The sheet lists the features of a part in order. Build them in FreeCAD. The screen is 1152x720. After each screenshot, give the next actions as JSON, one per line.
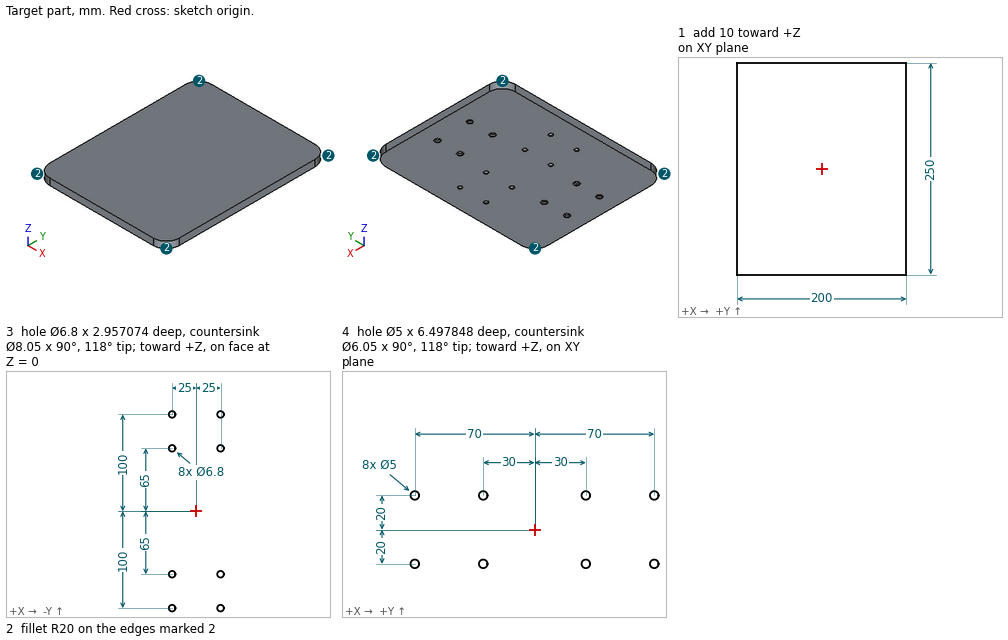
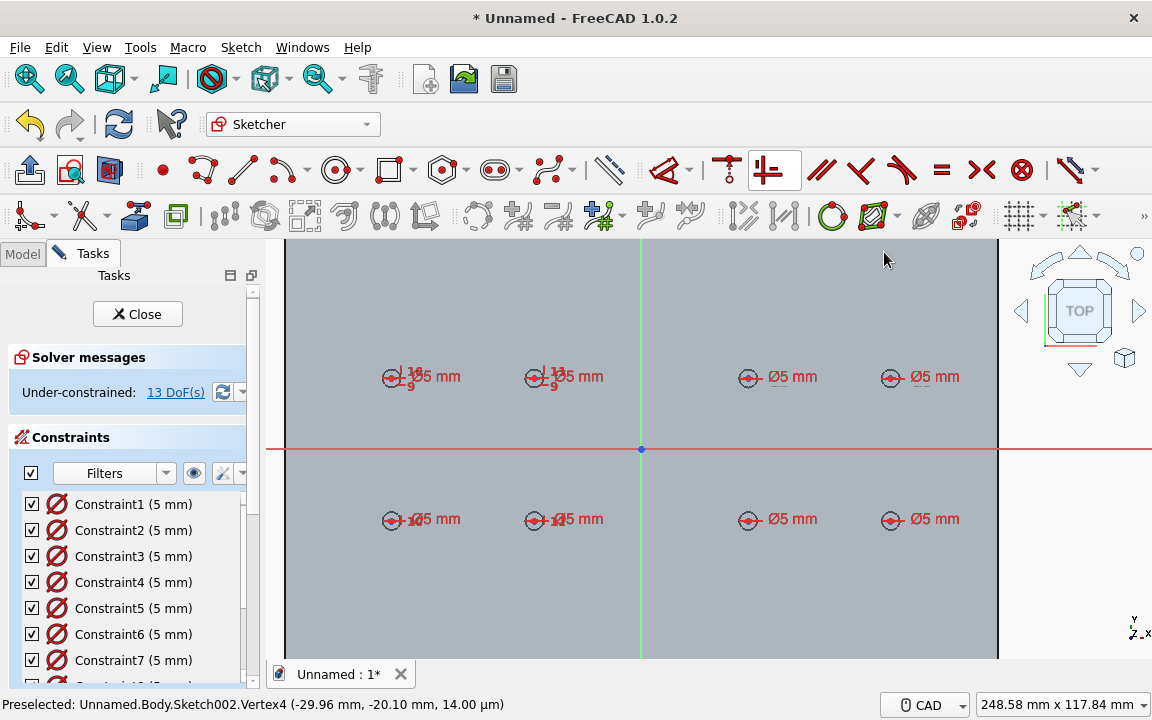
{"action": "left_click", "coordinate": [392, 521]}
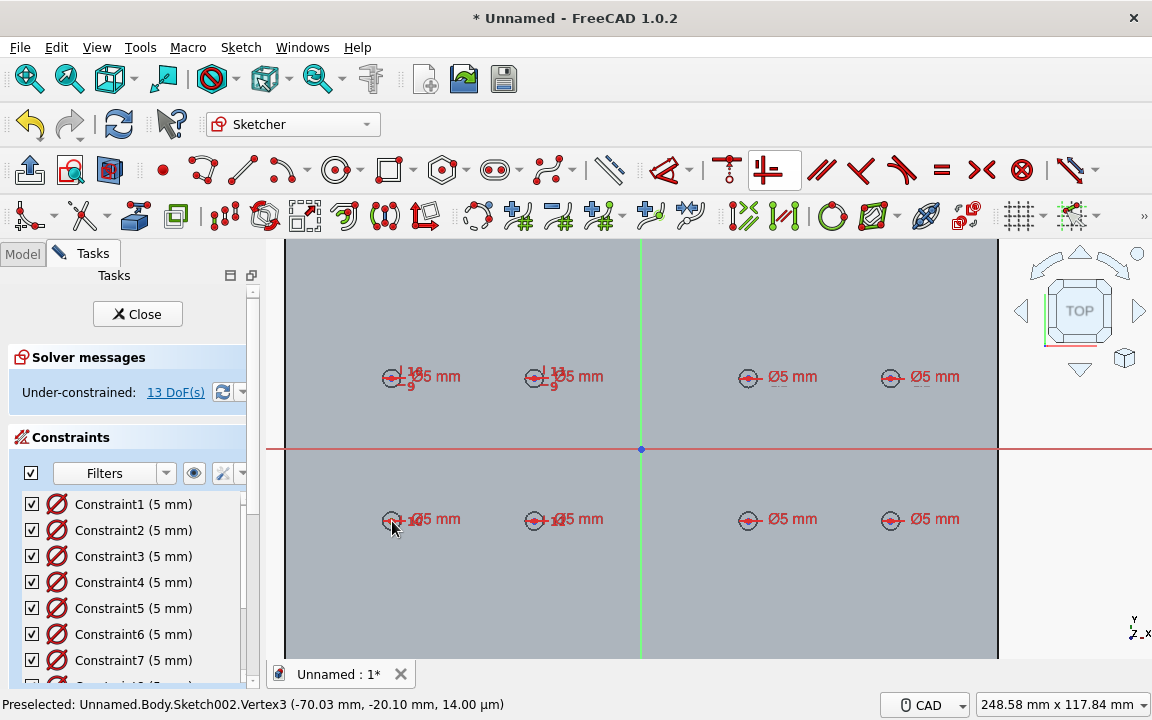
{"action": "left_click", "coordinate": [534, 521]}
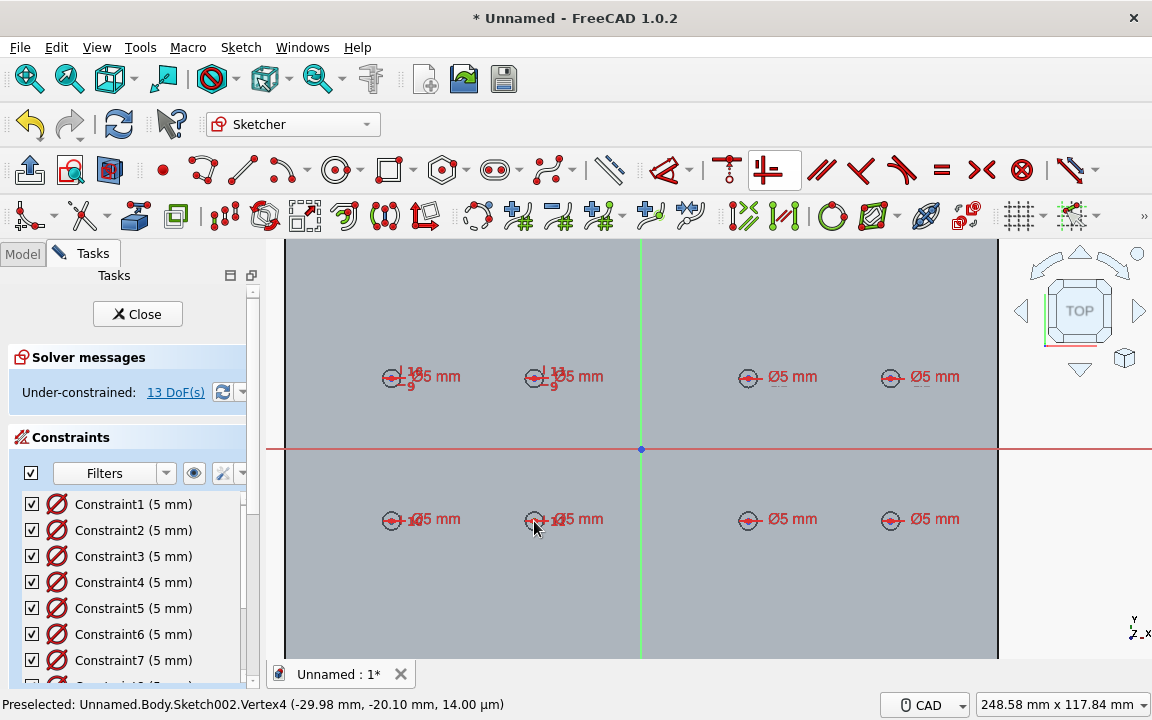
{"action": "key", "text": "h"}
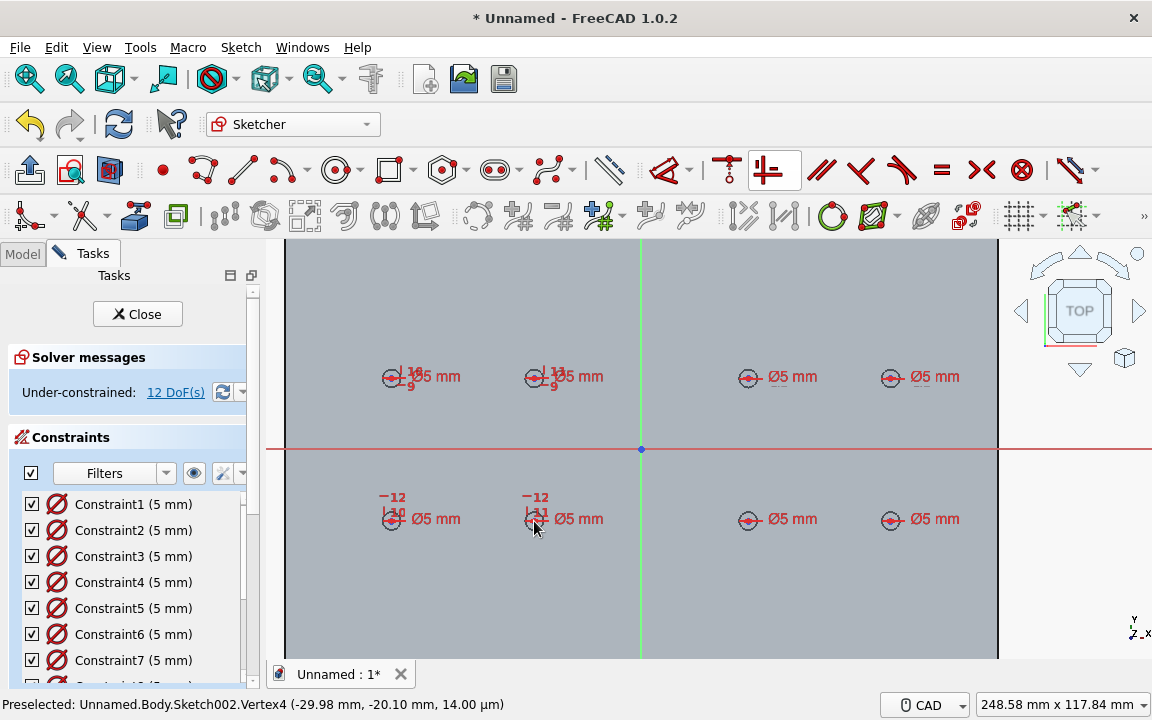
{"action": "left_click", "coordinate": [534, 378]}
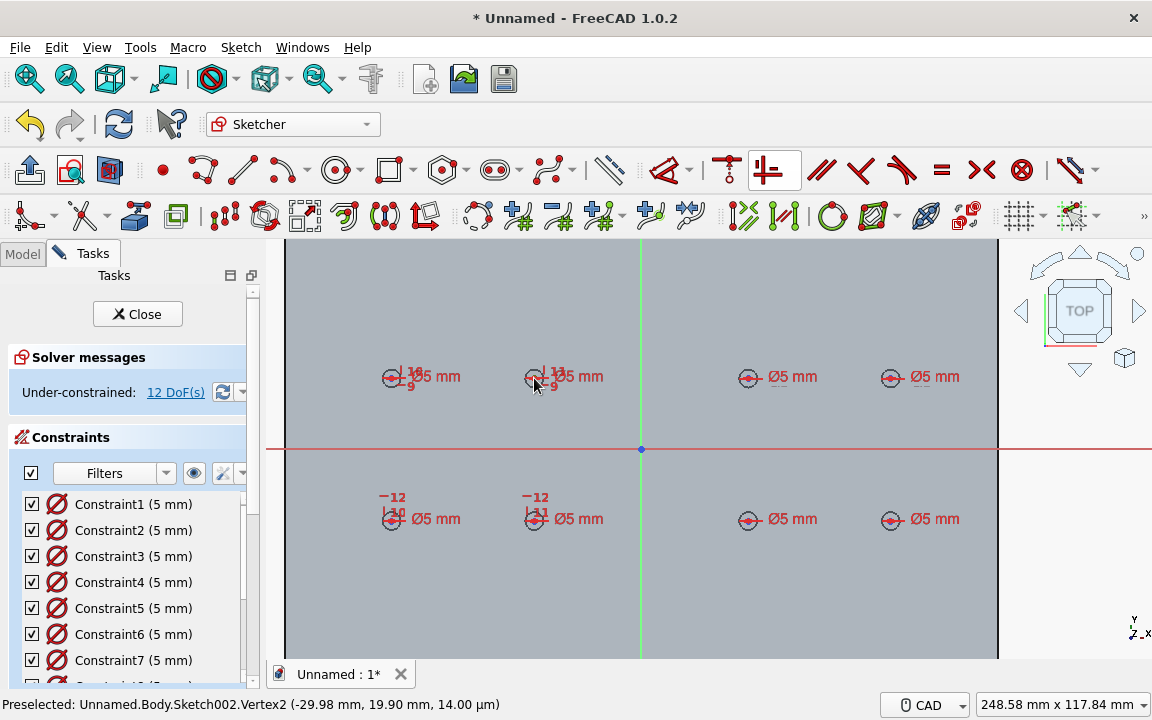
{"action": "left_click", "coordinate": [748, 379]}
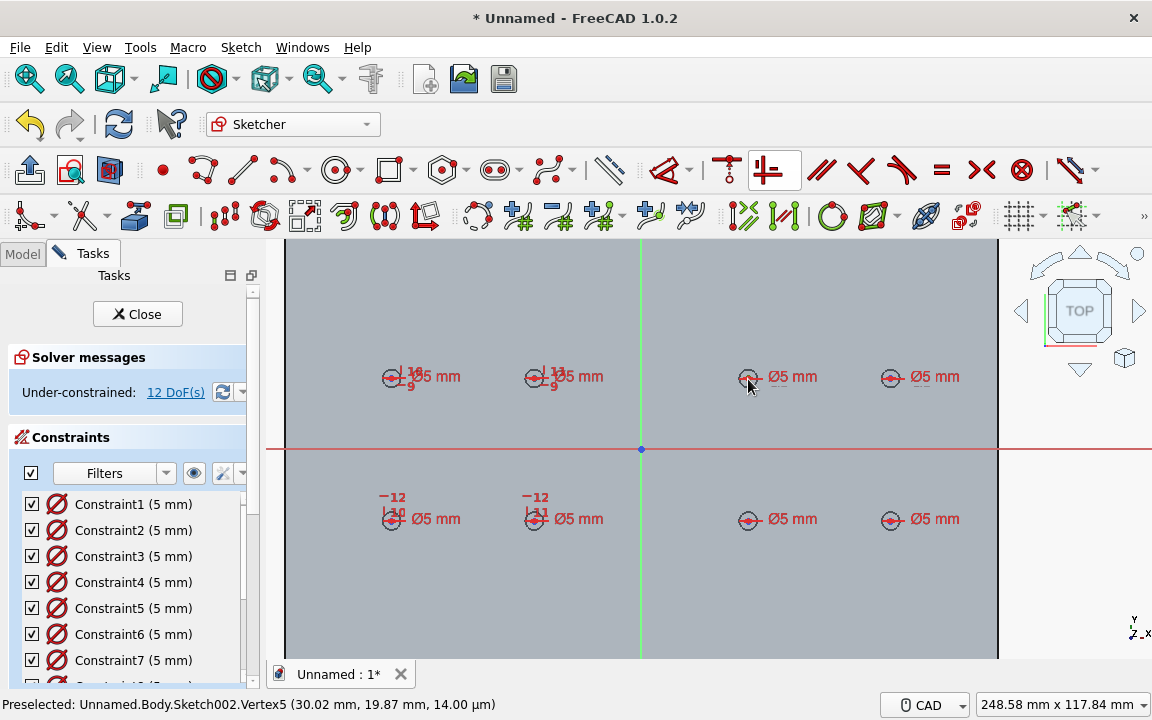
{"action": "key", "text": "h"}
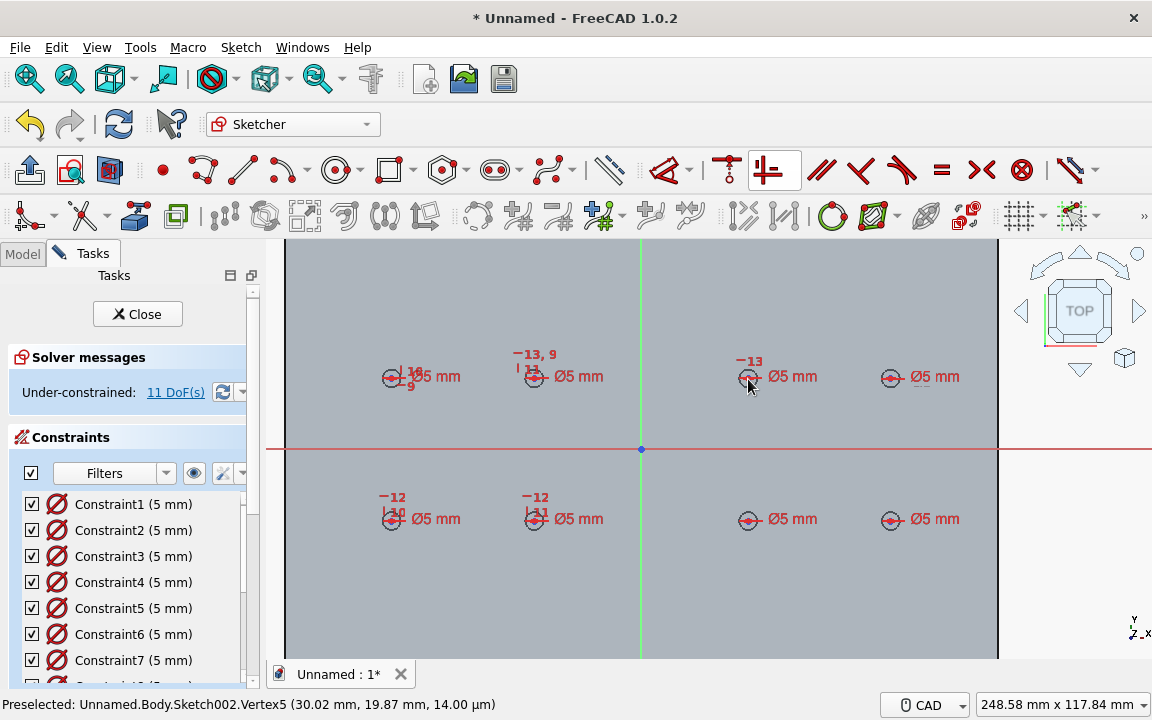
{"action": "left_click", "coordinate": [748, 378]}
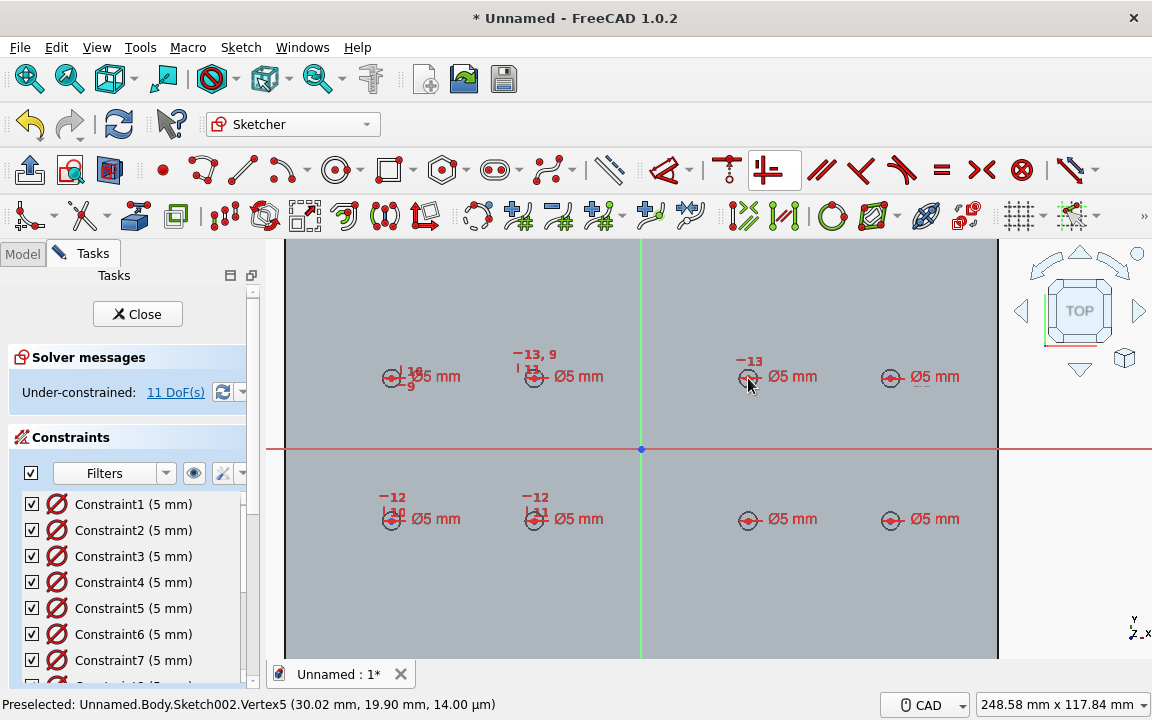
{"action": "left_click", "coordinate": [748, 521]}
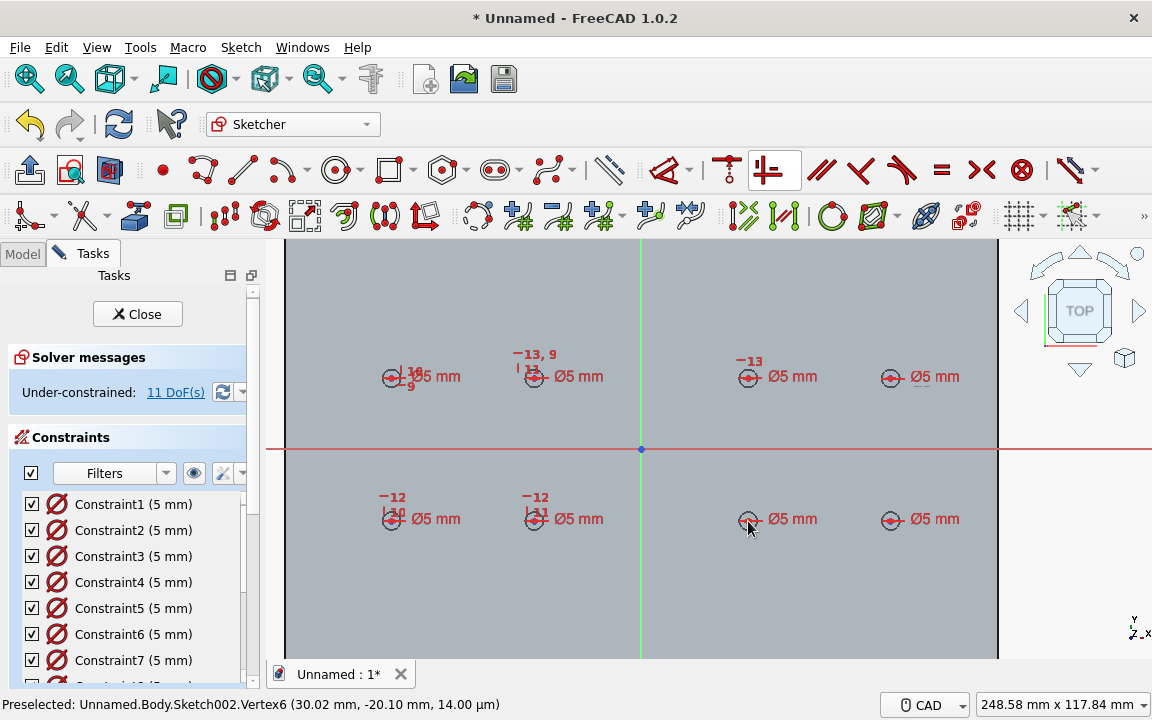
{"action": "key", "text": "v"}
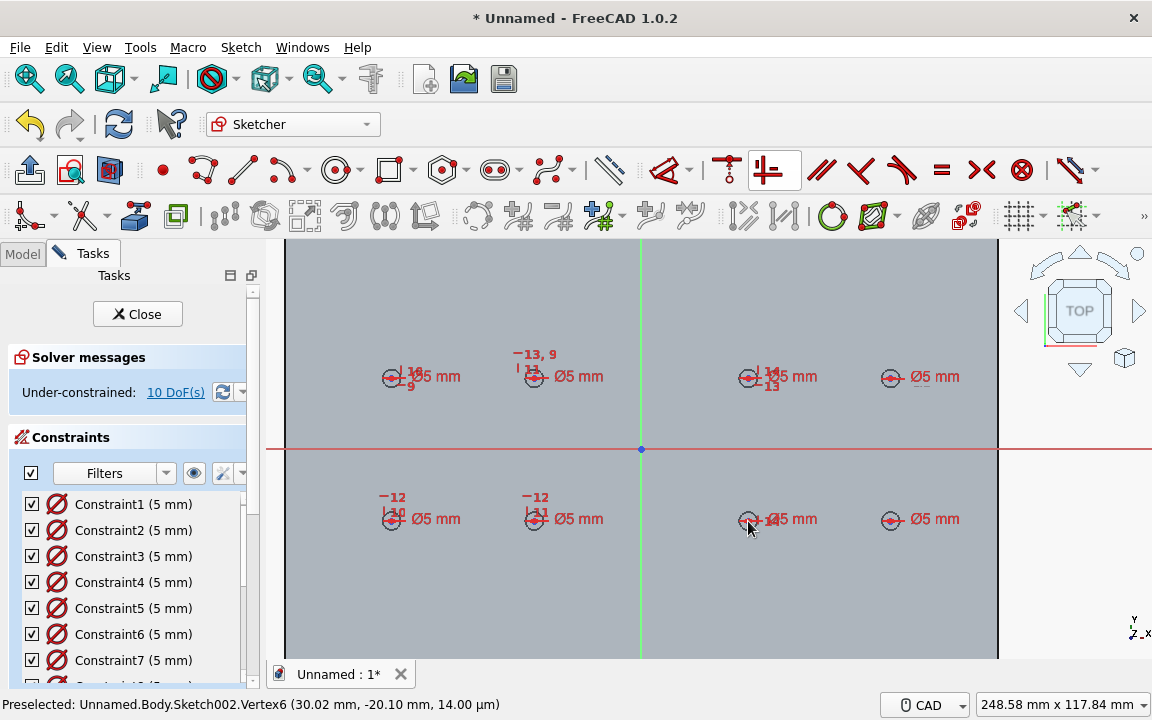
{"action": "left_click", "coordinate": [534, 521]}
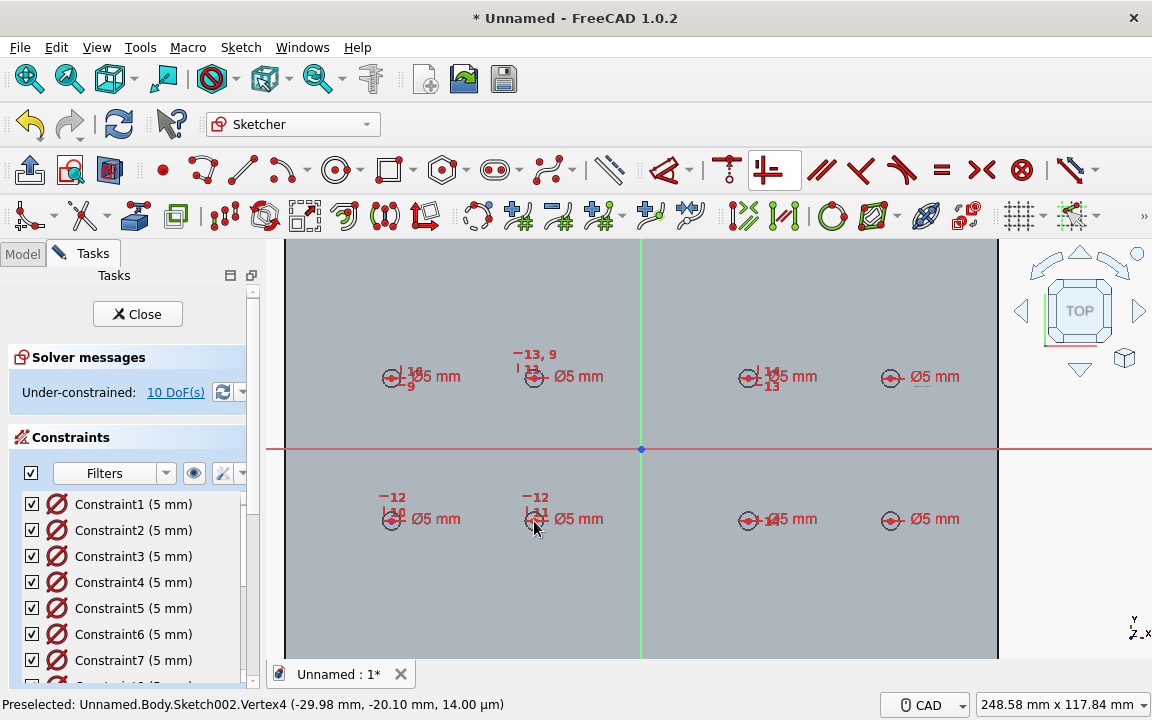
{"action": "left_click", "coordinate": [748, 521]}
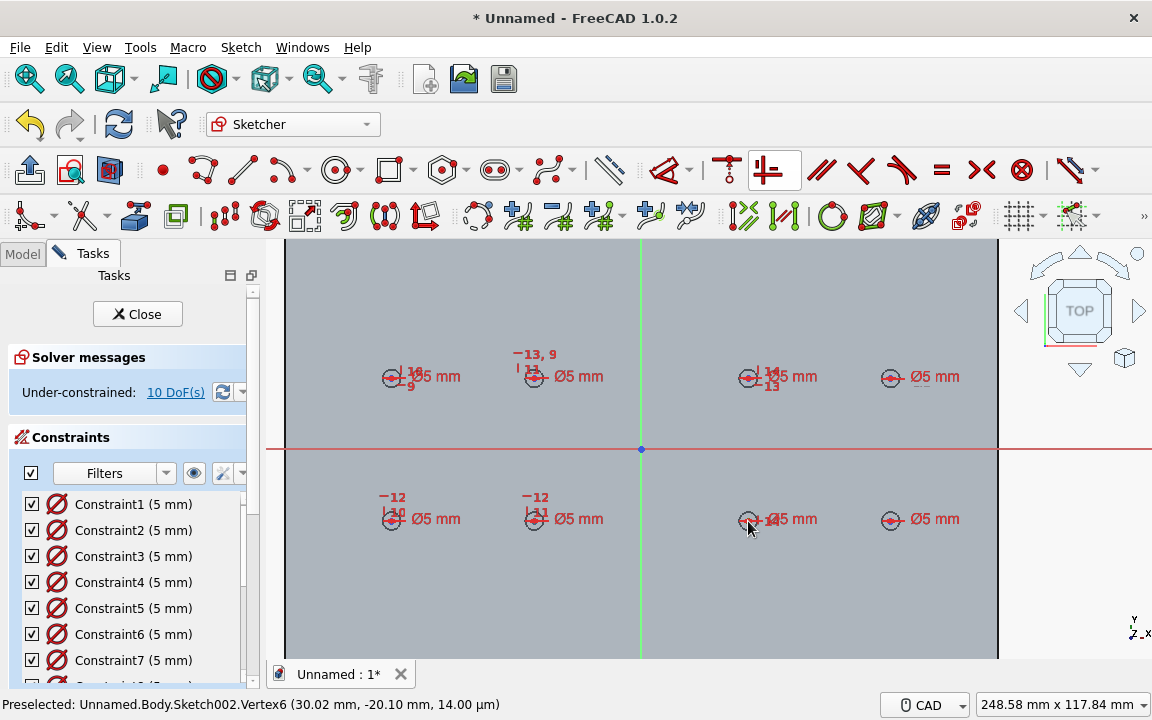
{"action": "key", "text": "h"}